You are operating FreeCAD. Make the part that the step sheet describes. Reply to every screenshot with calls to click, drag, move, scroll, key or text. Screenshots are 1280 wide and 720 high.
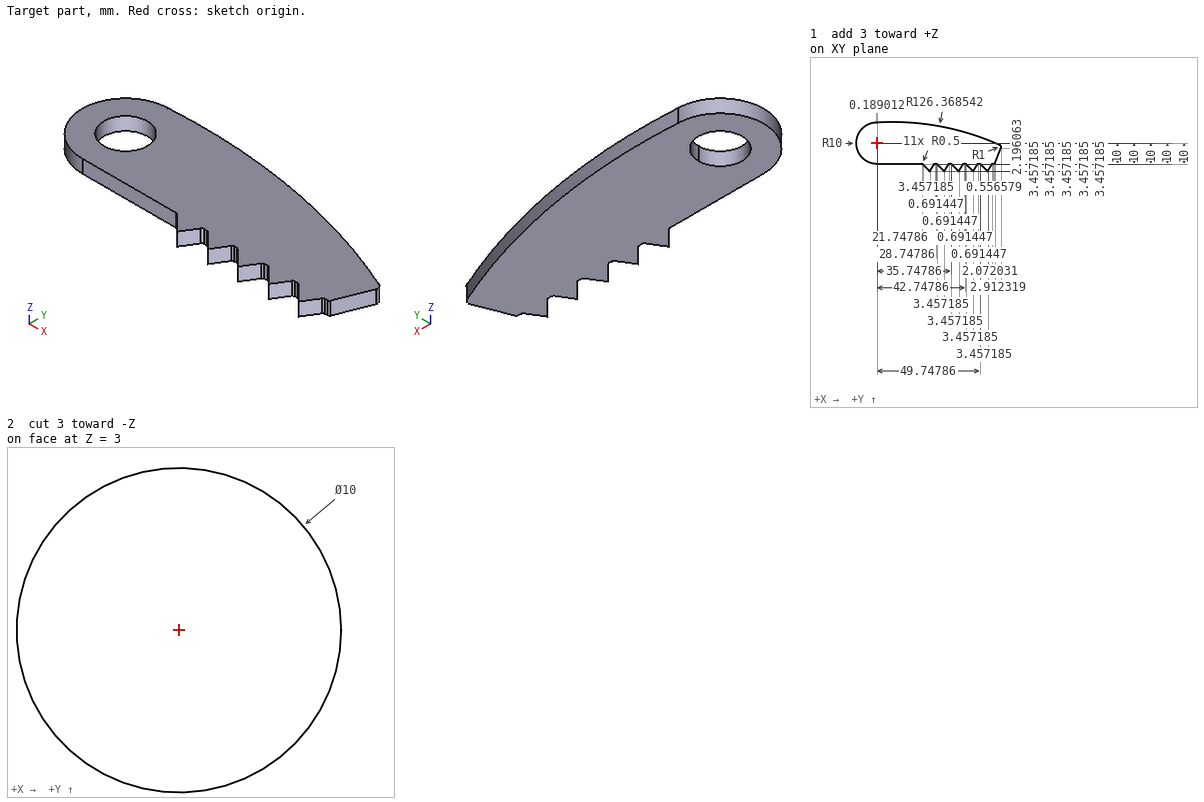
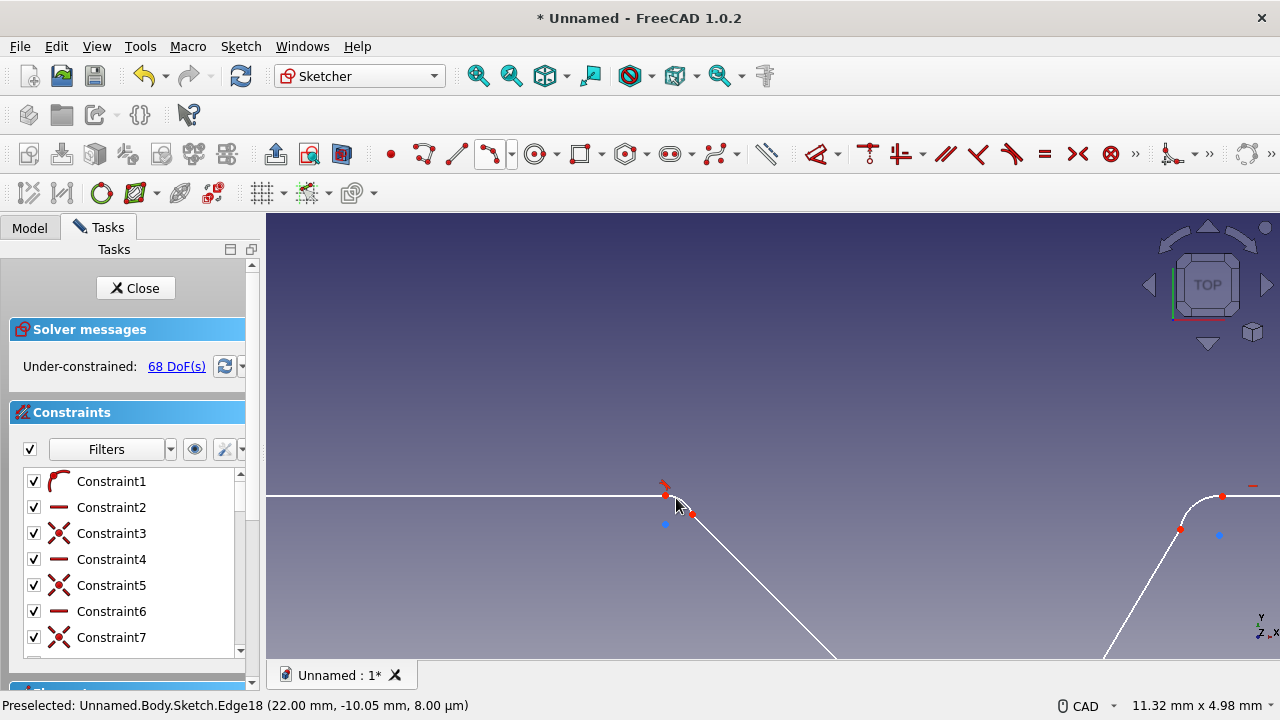
scroll(680, 503, down, 12)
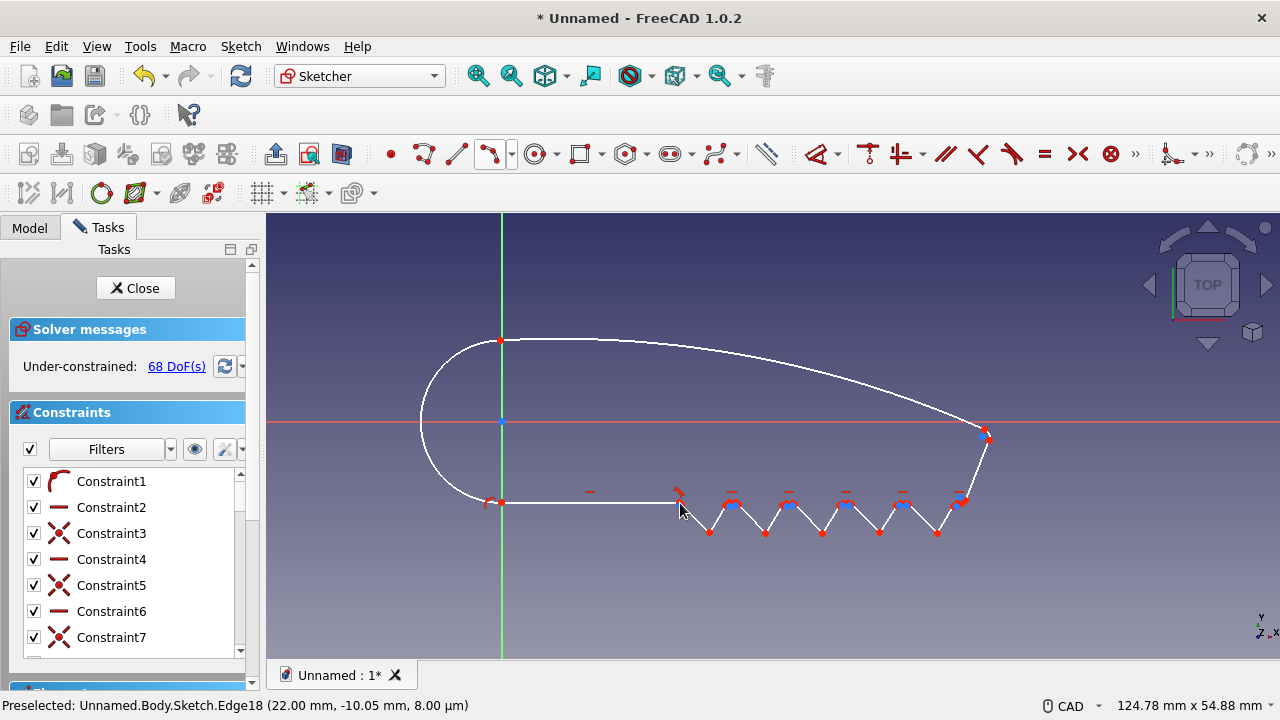
click(555, 503)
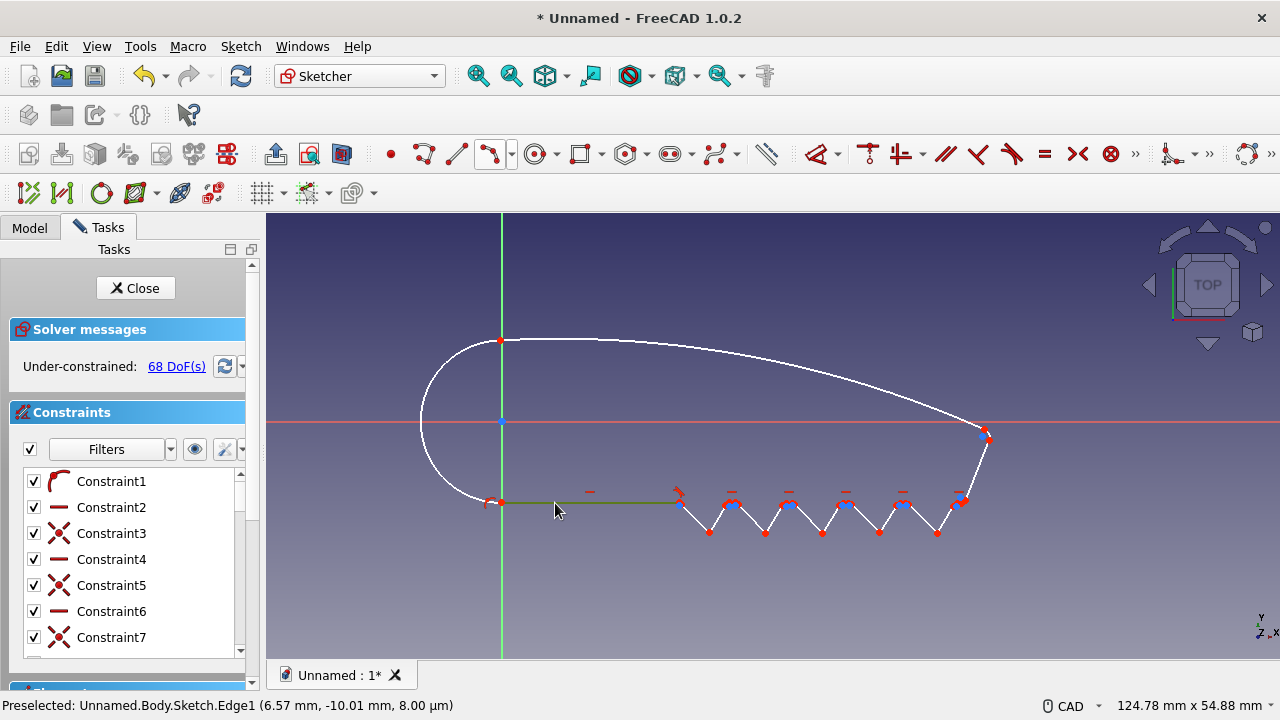
click(436, 375)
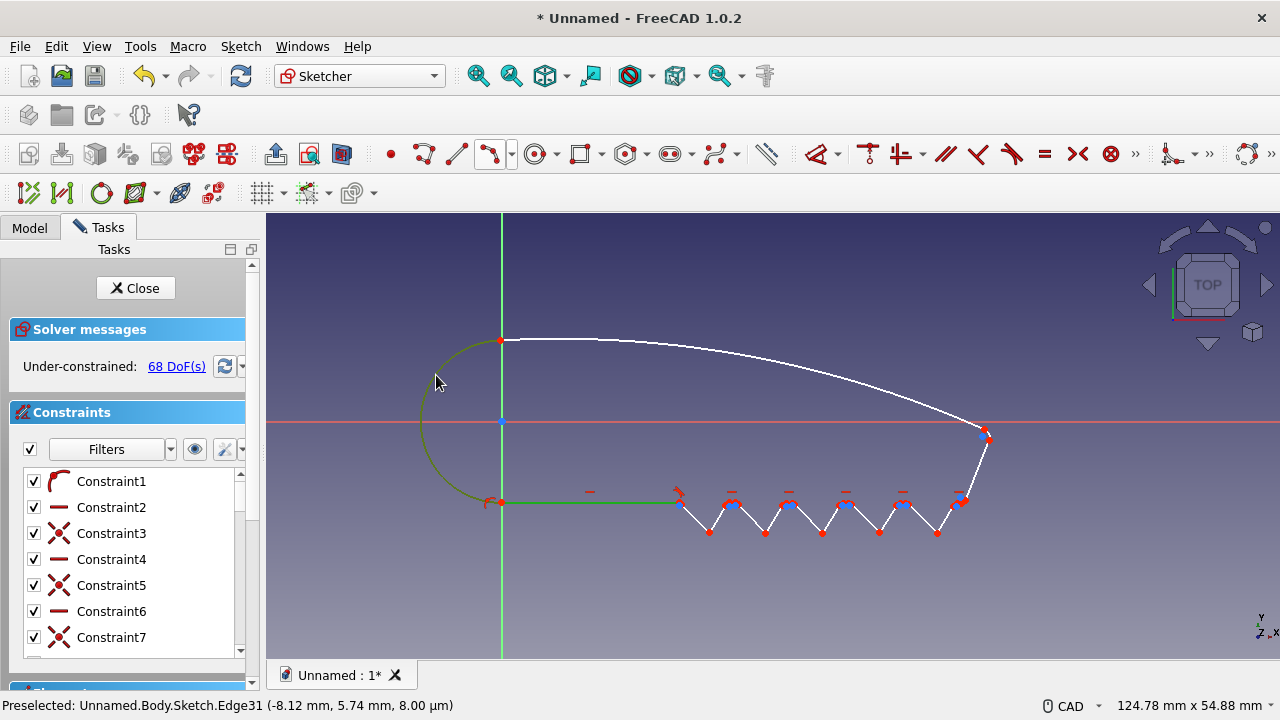
click(1012, 154)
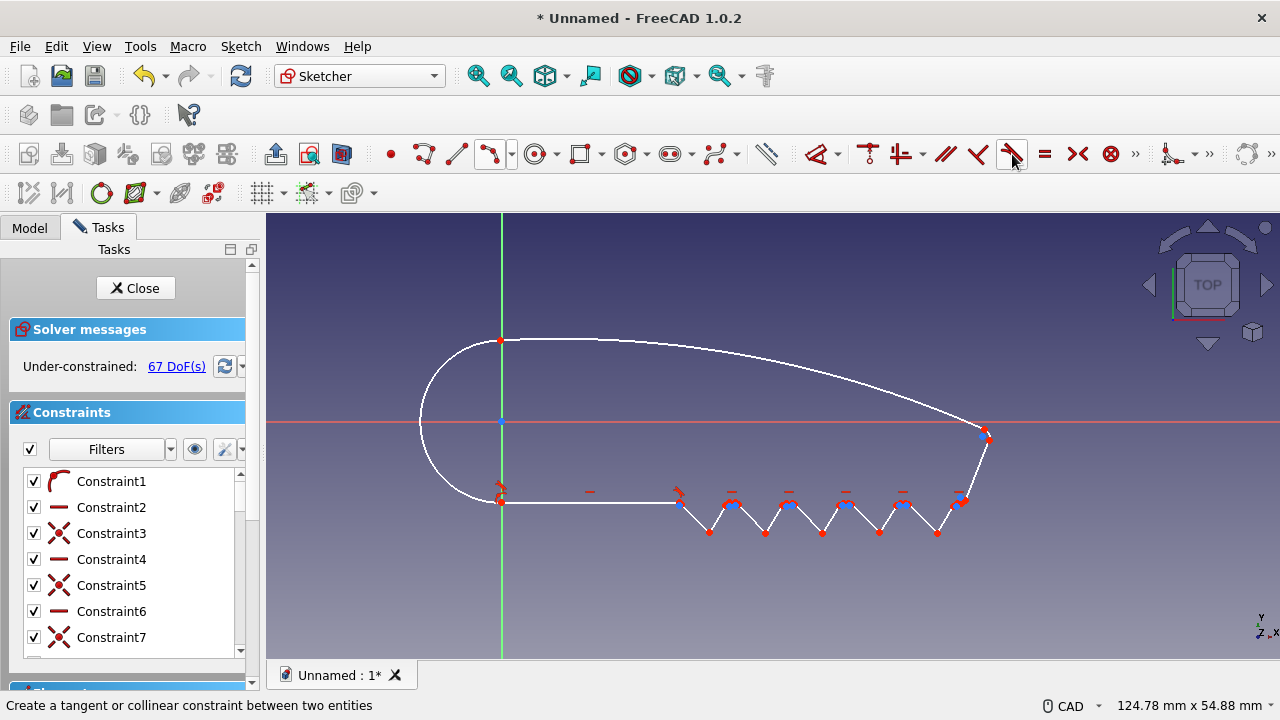
click(690, 513)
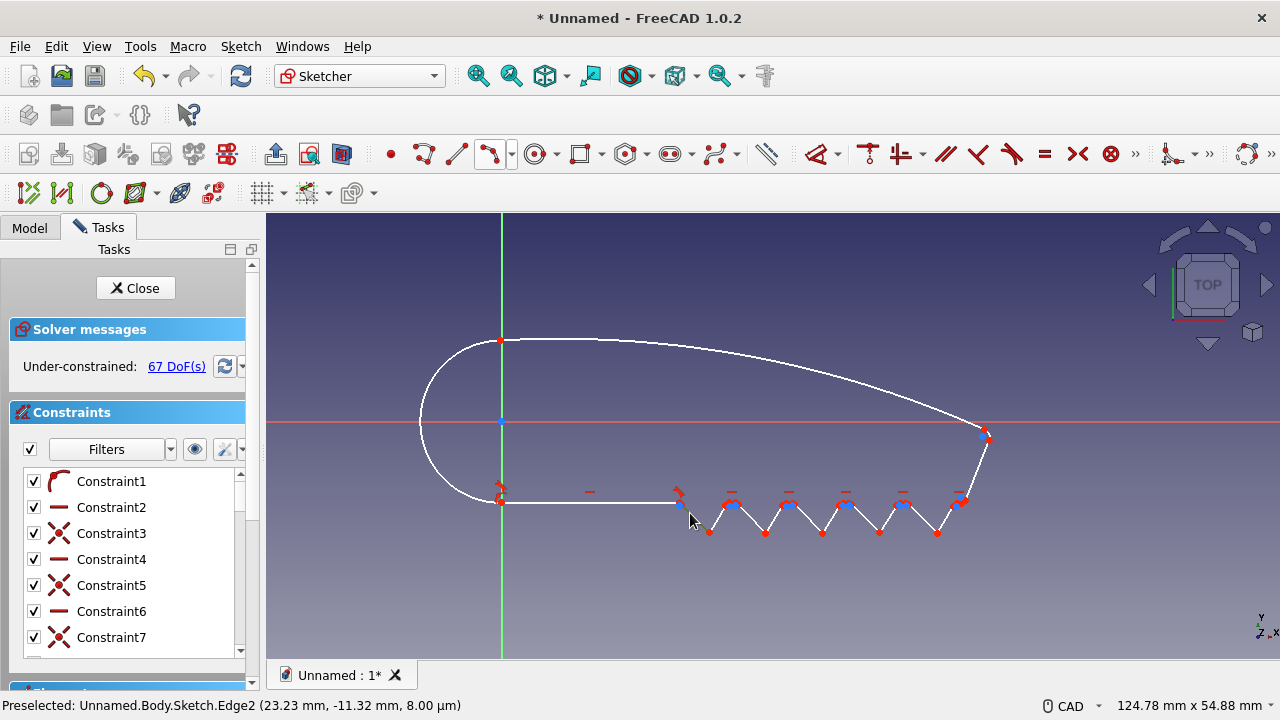
scroll(681, 503, up, 11)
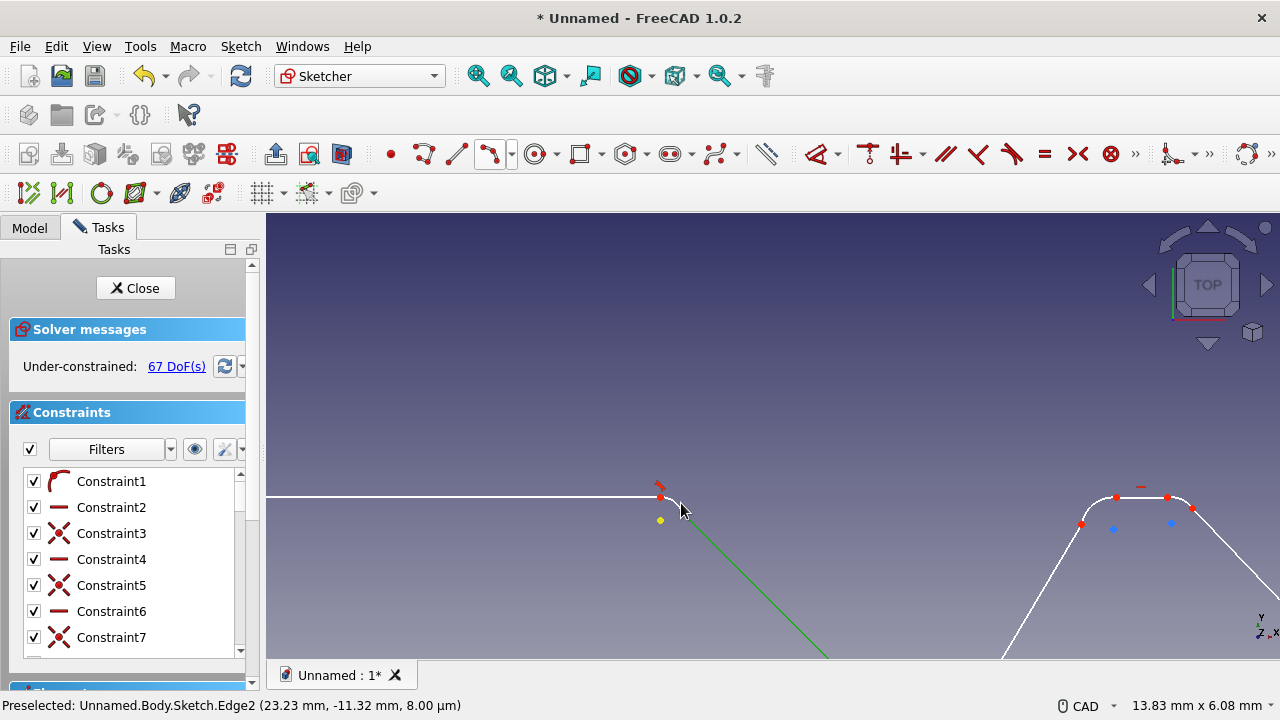
click(674, 501)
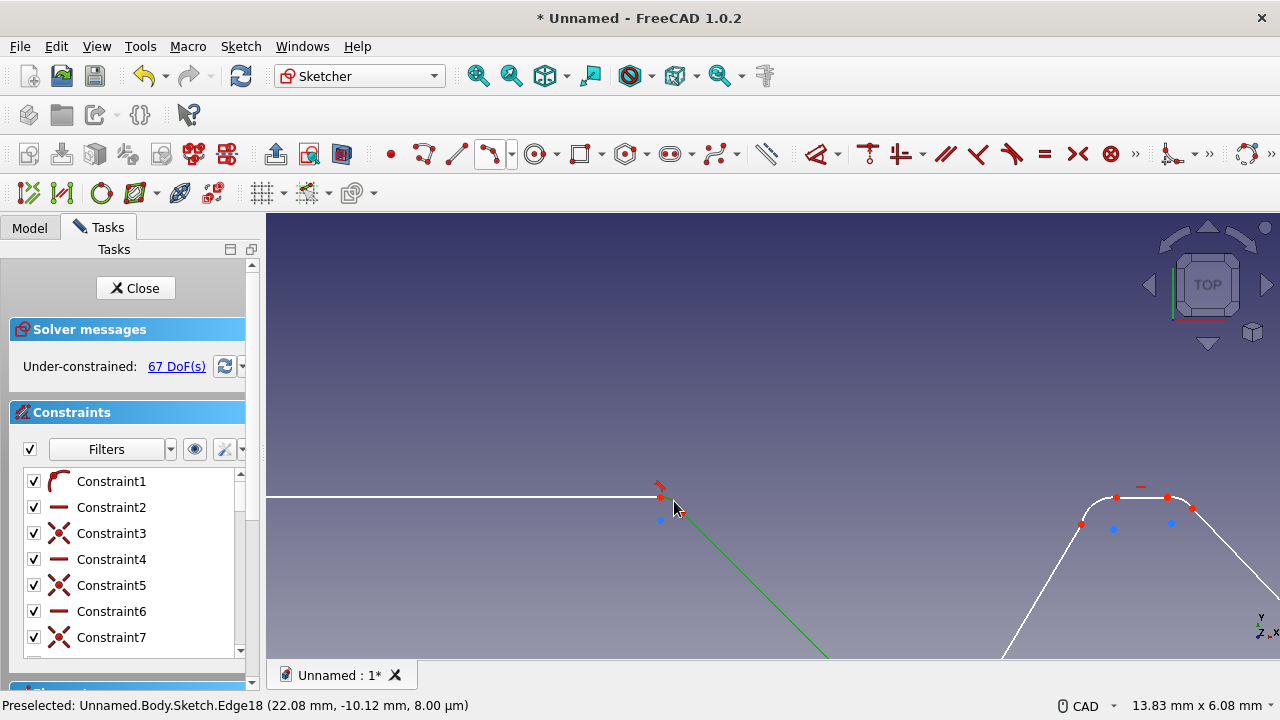
click(1012, 154)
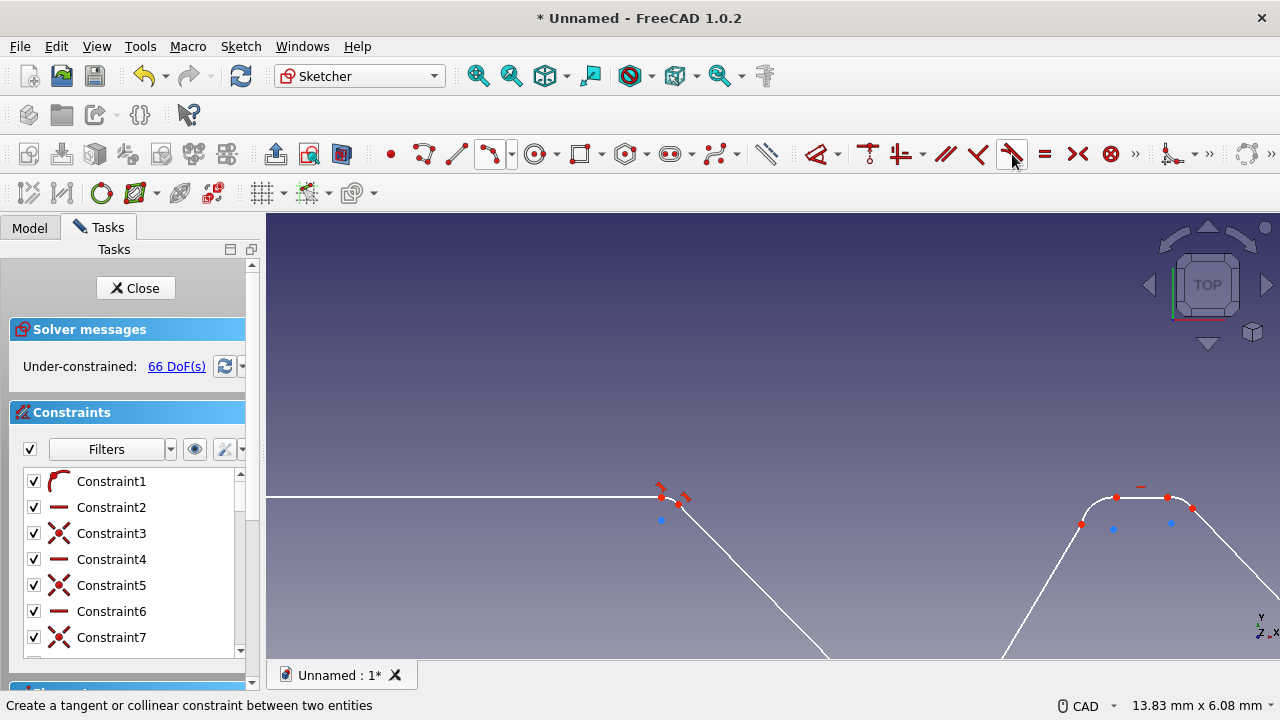
scroll(681, 503, down, 11)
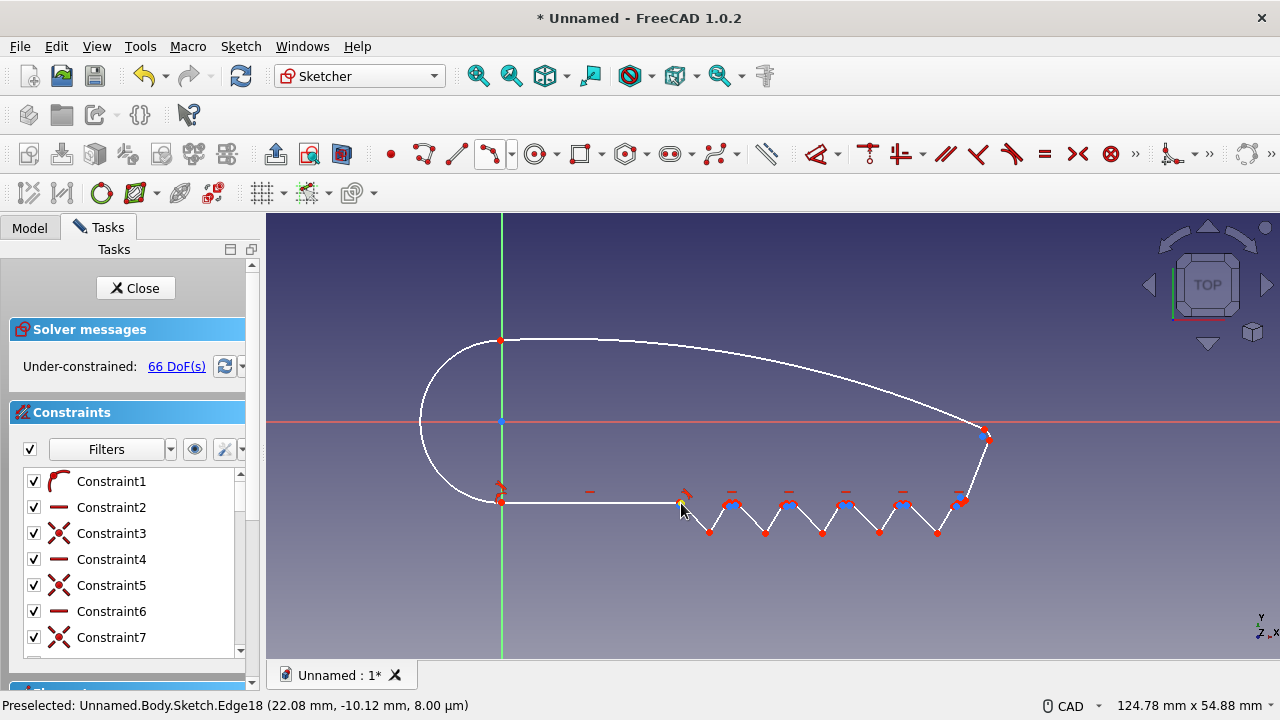
scroll(721, 514, up, 2)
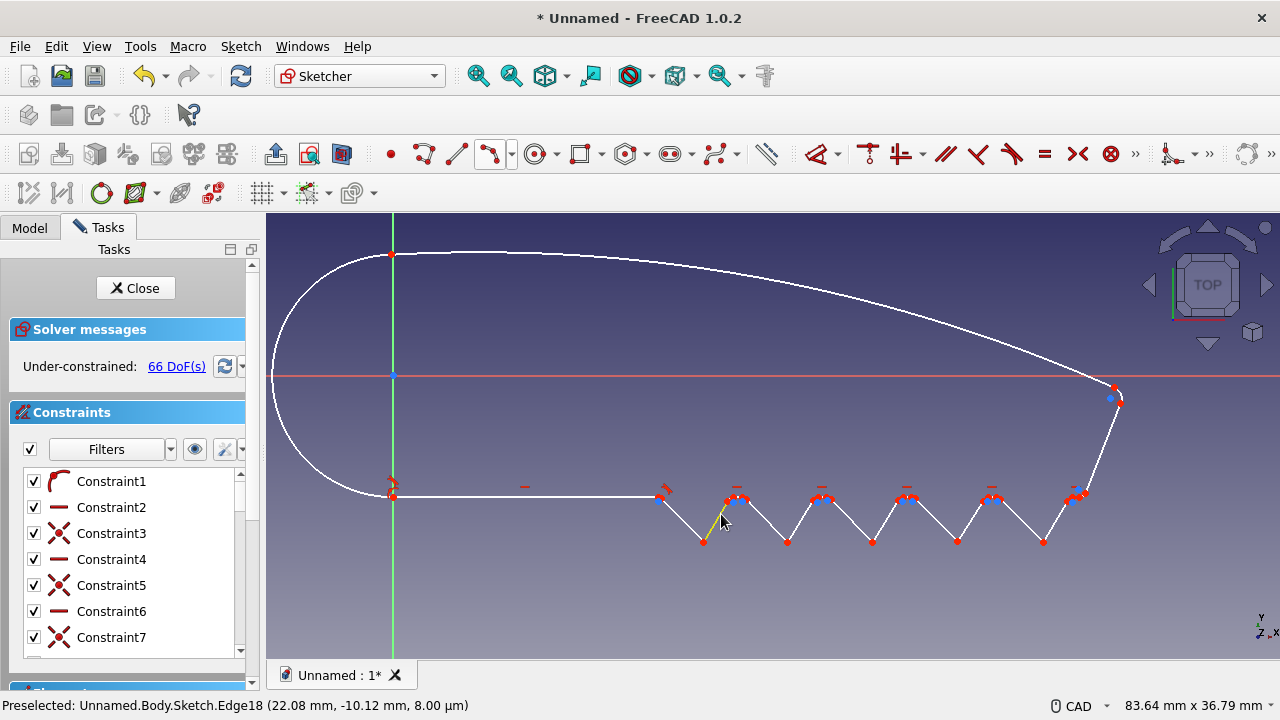
click(721, 514)